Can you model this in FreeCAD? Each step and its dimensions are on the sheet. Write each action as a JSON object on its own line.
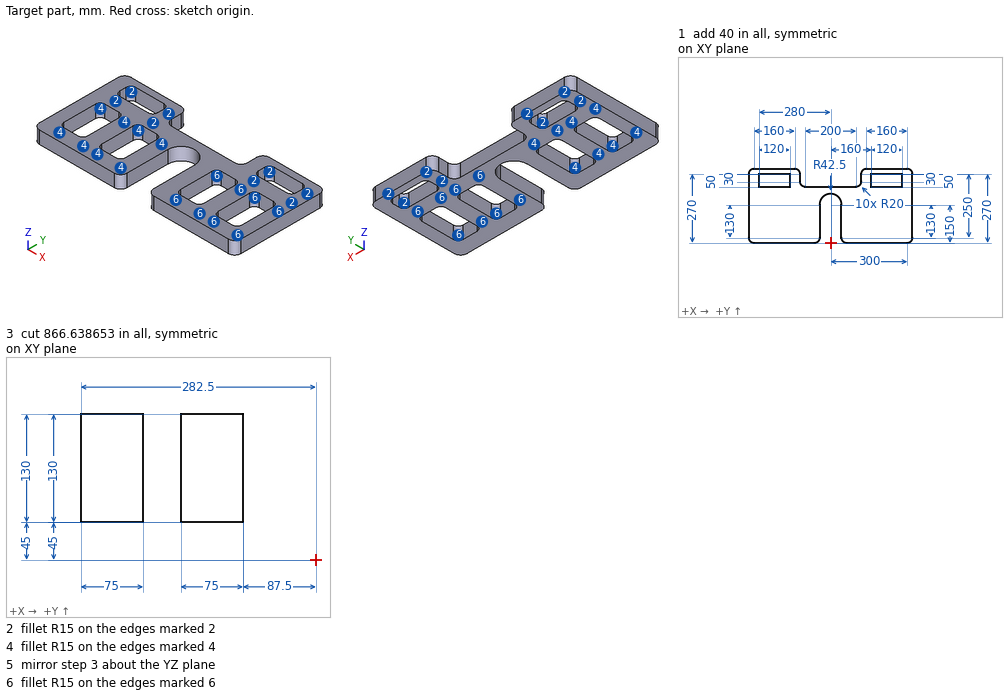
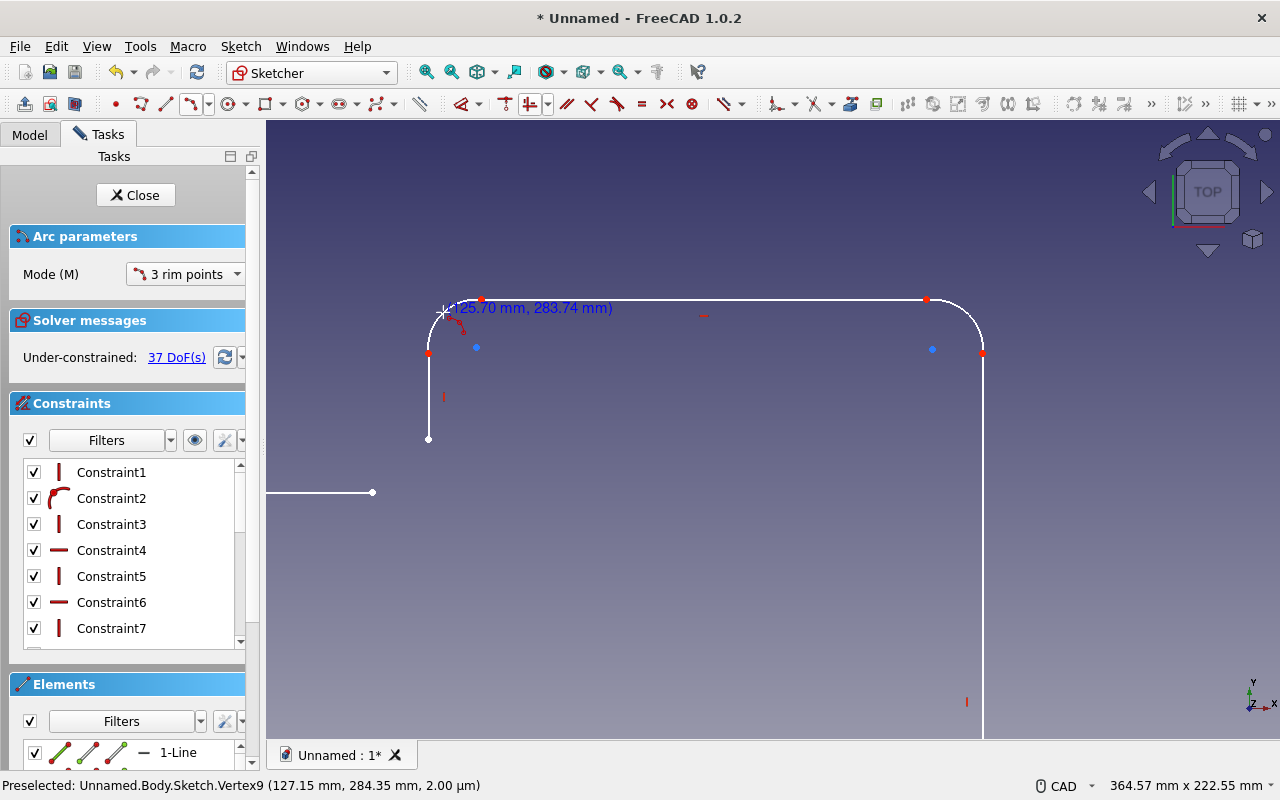
{"action": "left_click", "coordinate": [429, 439]}
{"action": "left_click", "coordinate": [372, 493]}
{"action": "left_click", "coordinate": [411, 474]}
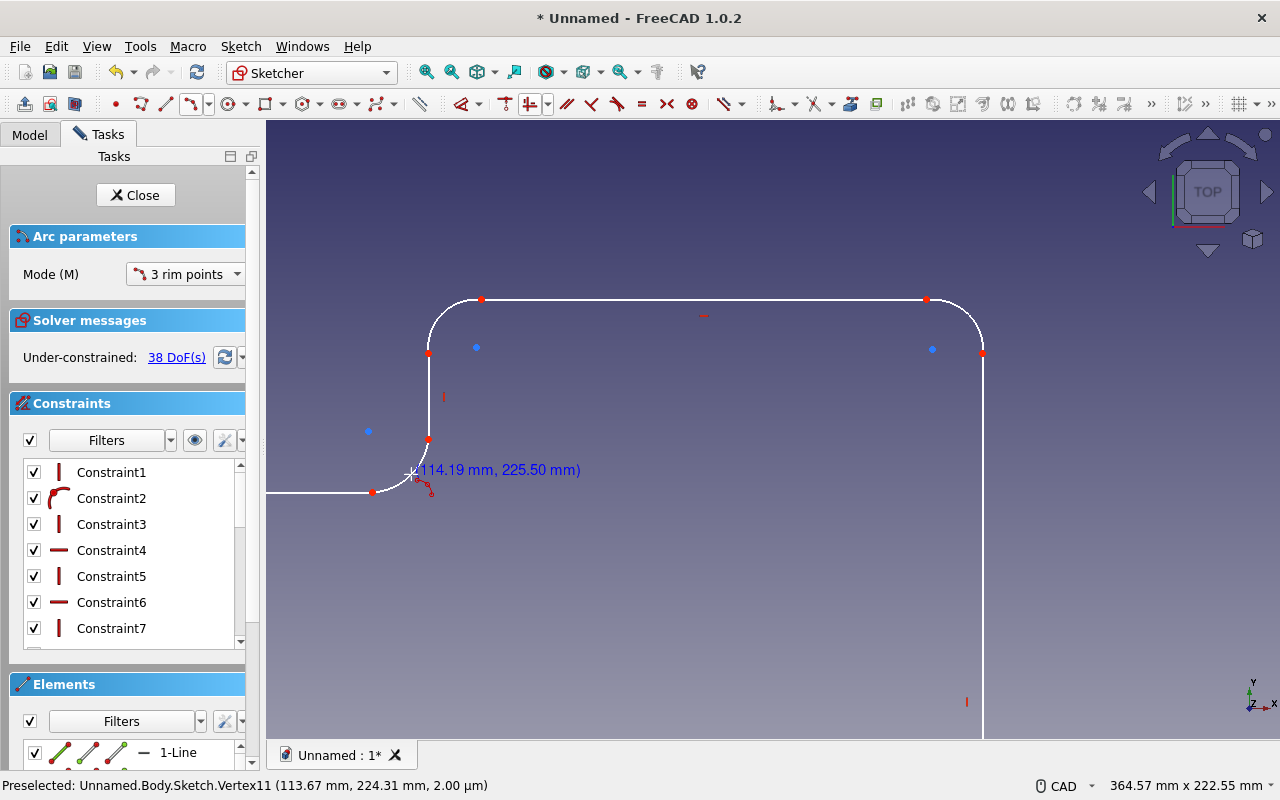
{"action": "scroll", "coordinate": [968, 313], "scroll_direction": "down", "scroll_amount": 6}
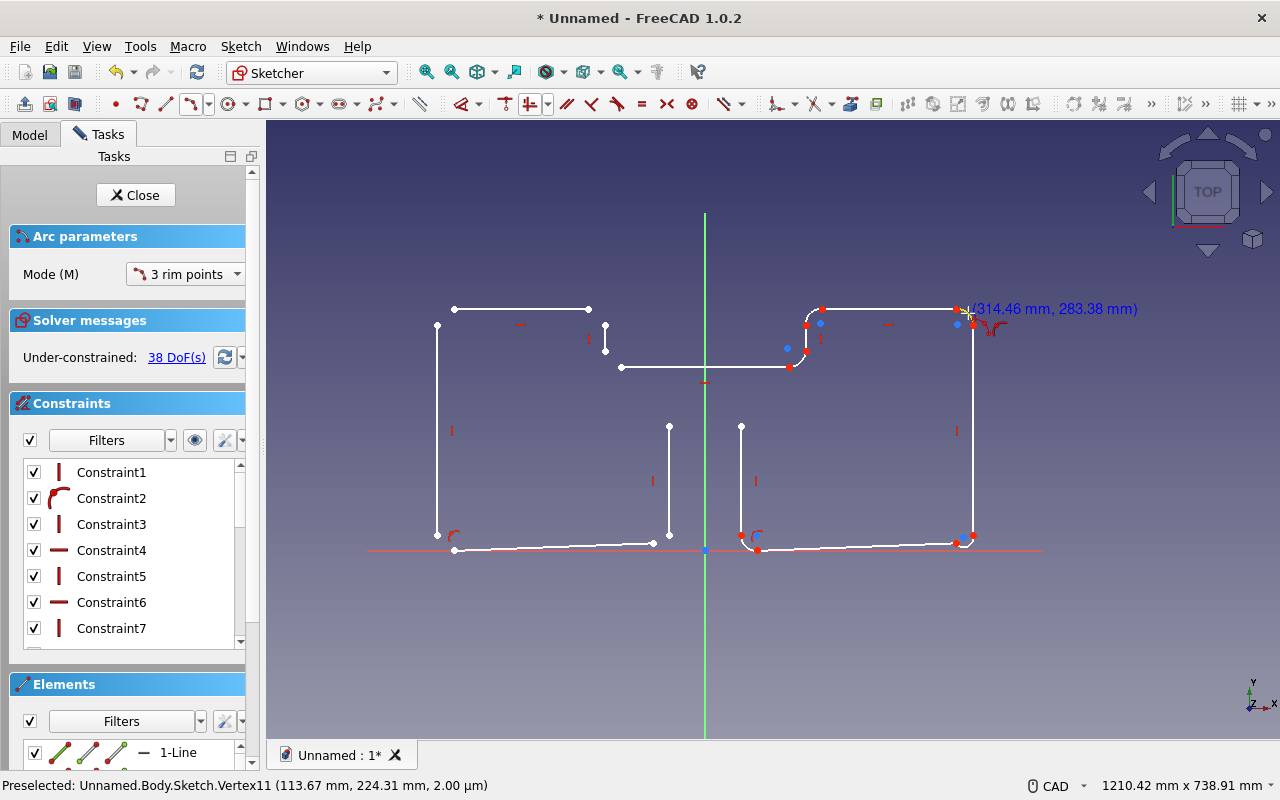
{"action": "left_click", "coordinate": [621, 367]}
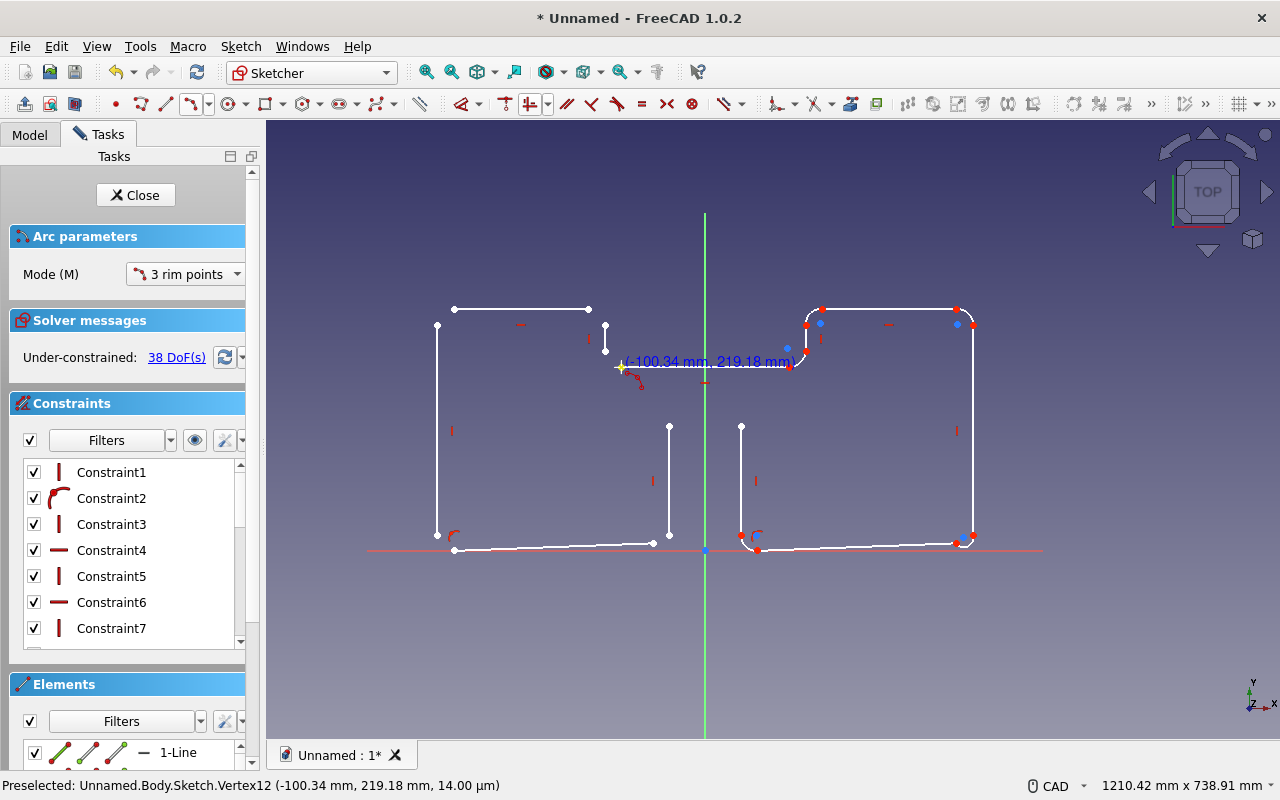
{"action": "scroll", "coordinate": [605, 350], "scroll_direction": "up", "scroll_amount": 2}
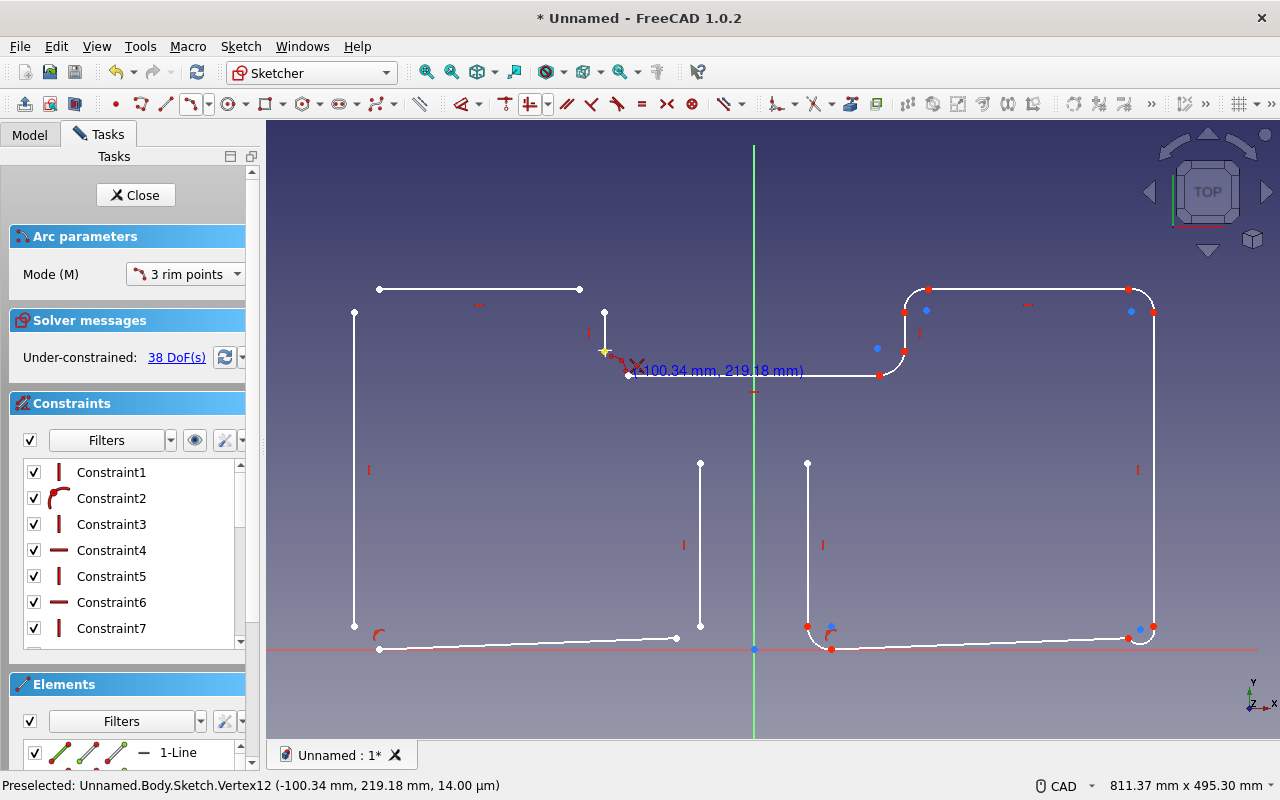
{"action": "left_click", "coordinate": [605, 352]}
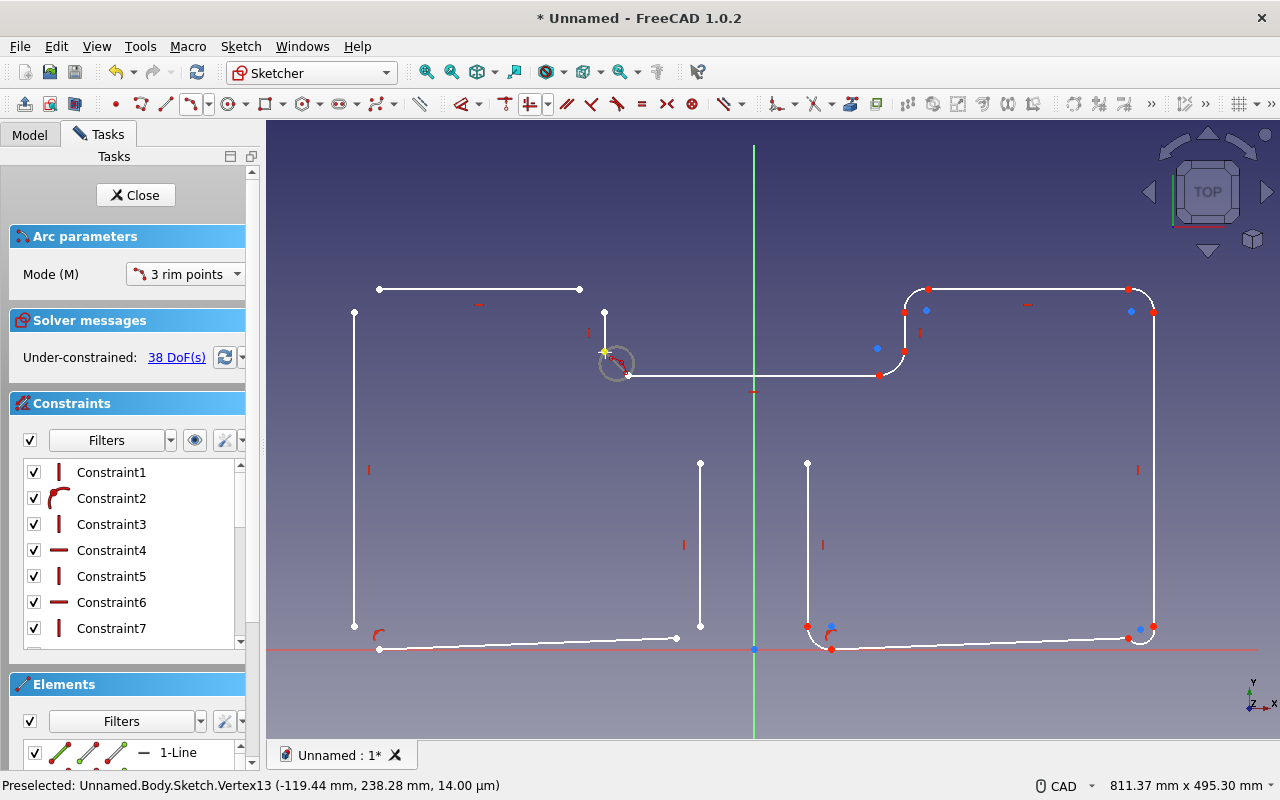
{"action": "scroll", "coordinate": [611, 367], "scroll_direction": "up", "scroll_amount": 4}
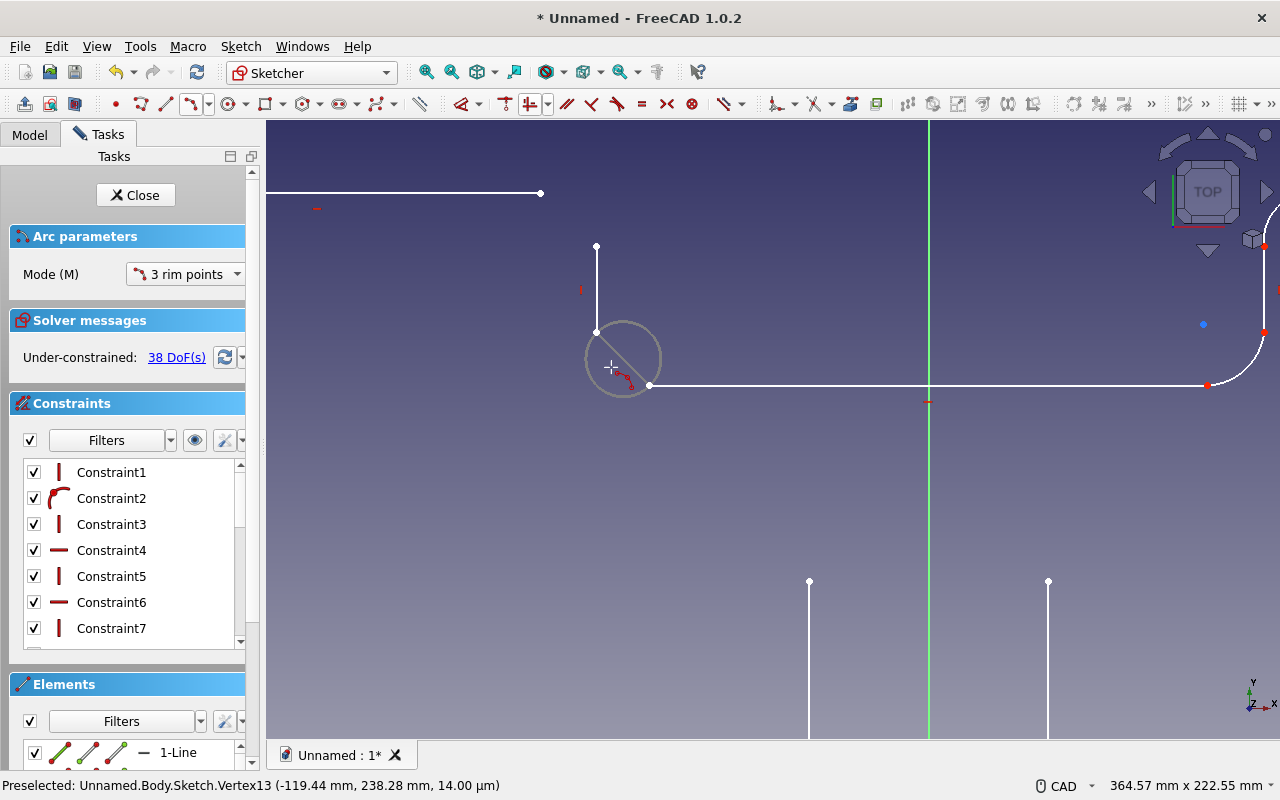
{"action": "left_click", "coordinate": [612, 367]}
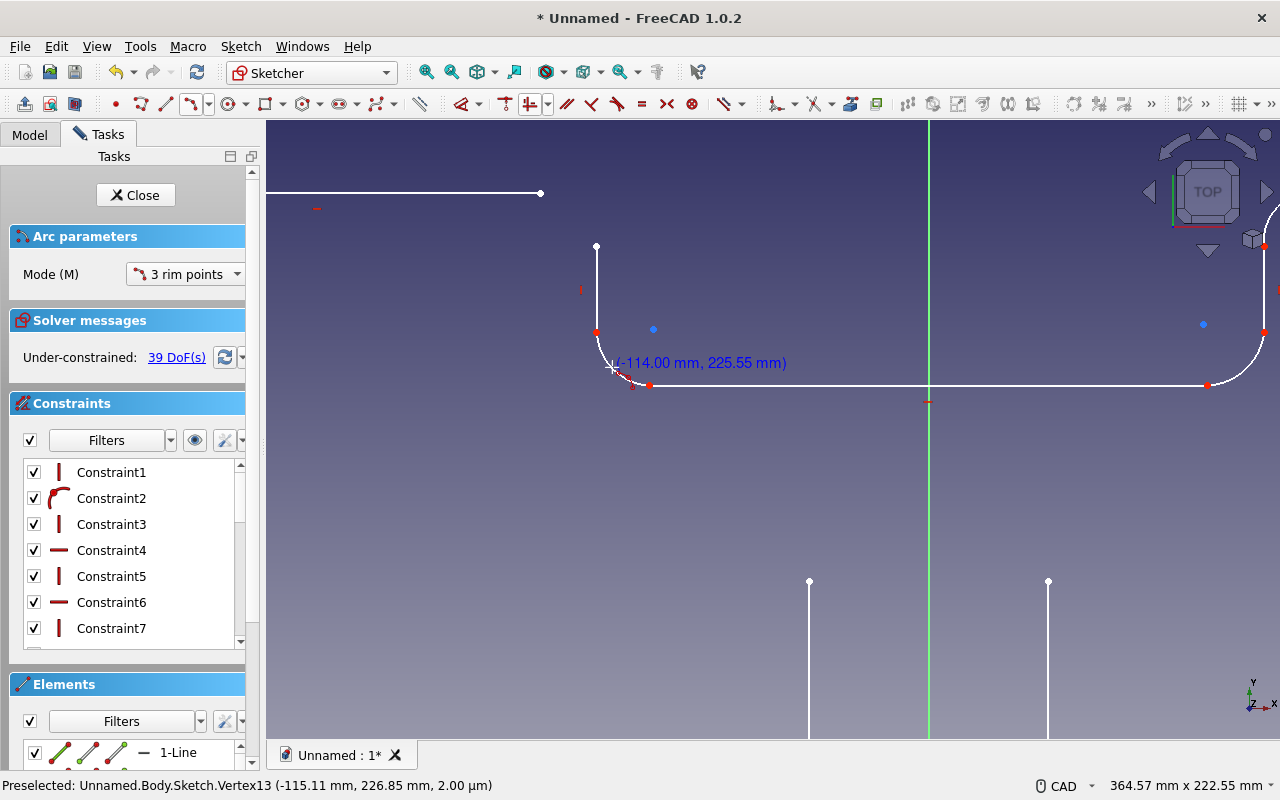
{"action": "left_click", "coordinate": [597, 246]}
{"action": "left_click", "coordinate": [540, 193]}
{"action": "left_click", "coordinate": [579, 205]}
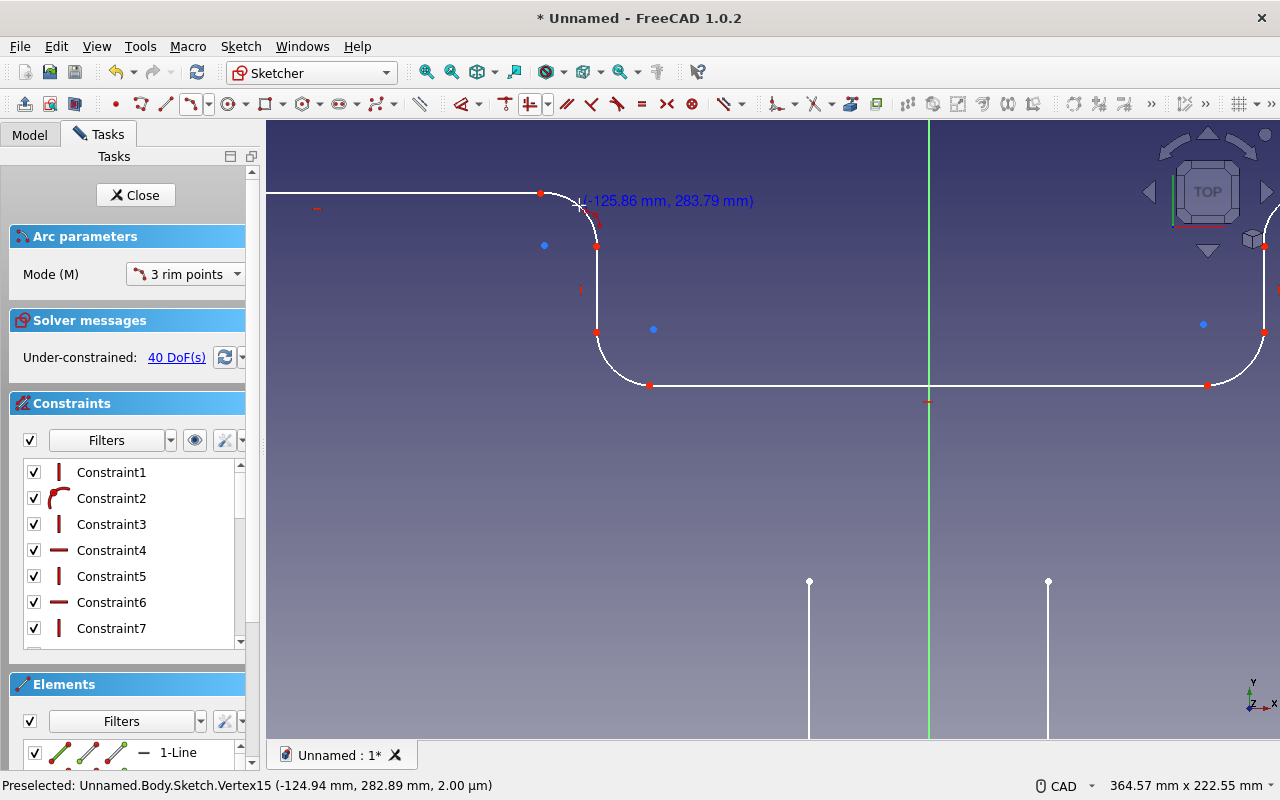
{"action": "scroll", "coordinate": [608, 359], "scroll_direction": "down", "scroll_amount": 6}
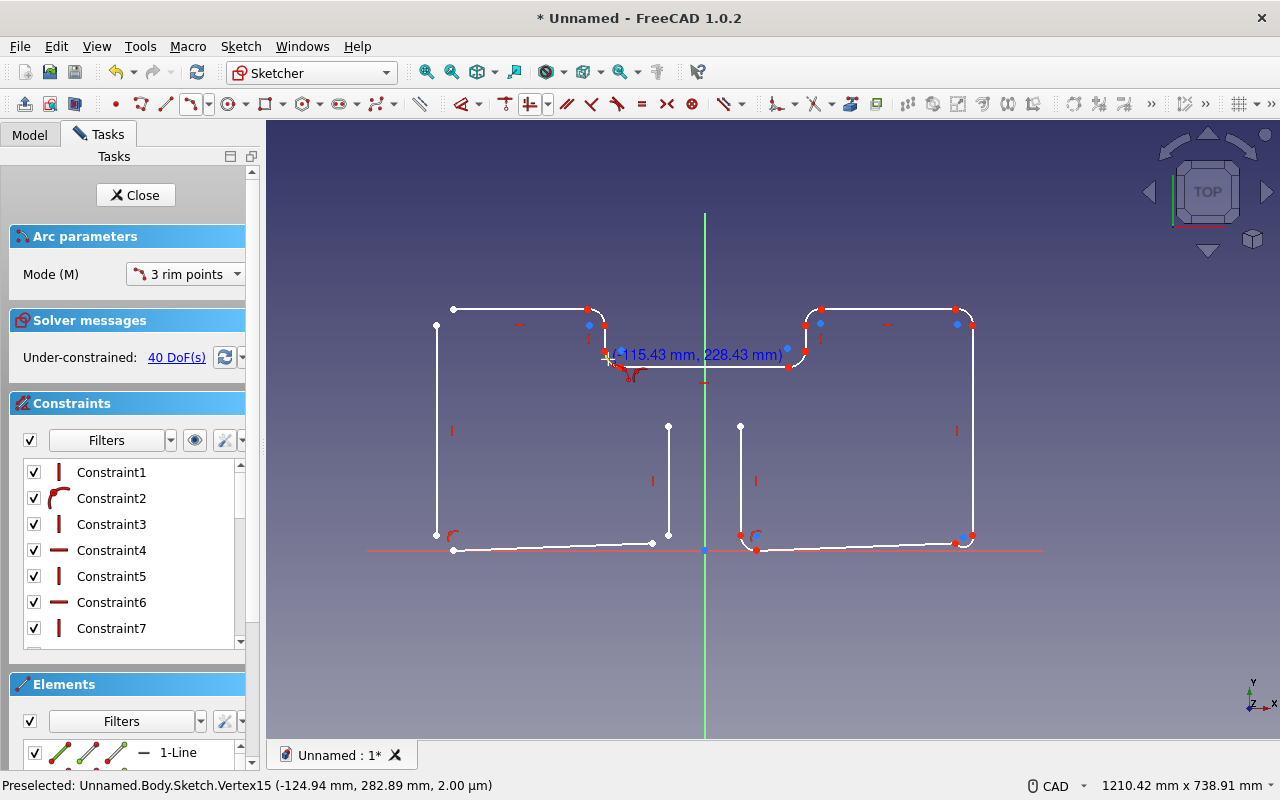
{"action": "left_click", "coordinate": [454, 309]}
{"action": "left_click", "coordinate": [437, 325]}